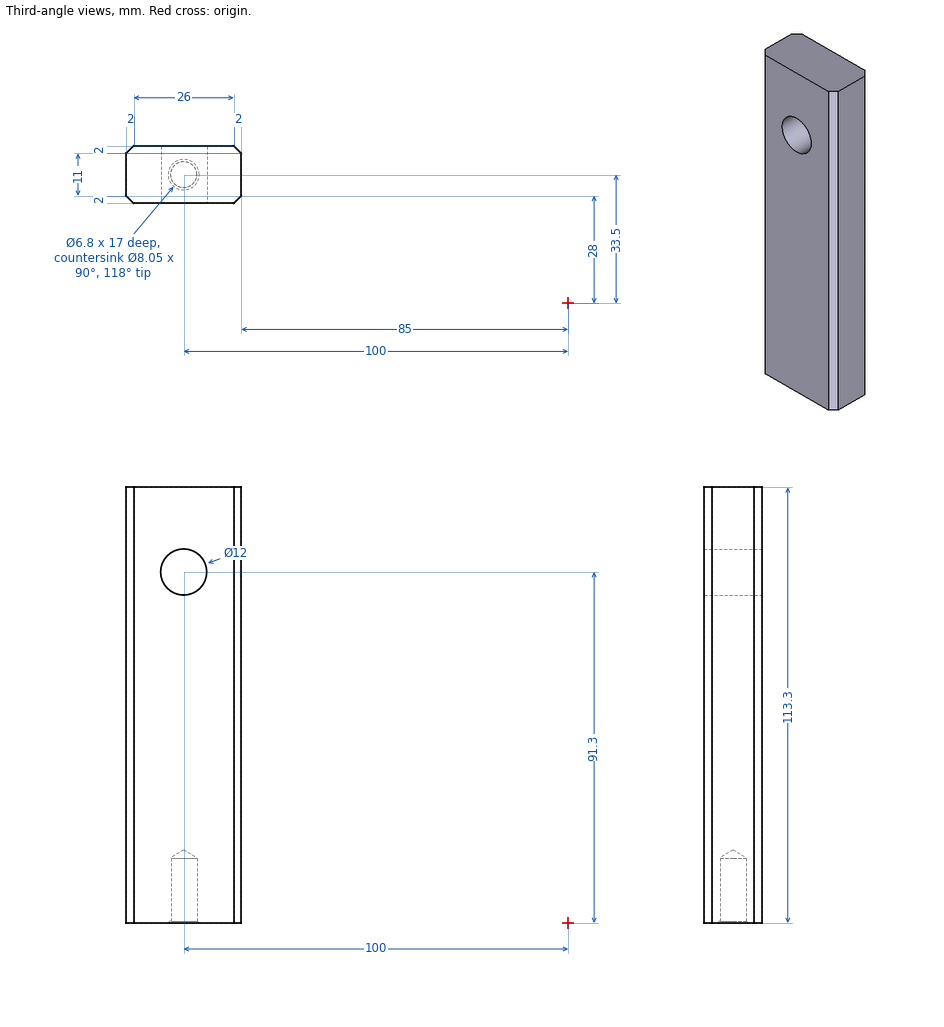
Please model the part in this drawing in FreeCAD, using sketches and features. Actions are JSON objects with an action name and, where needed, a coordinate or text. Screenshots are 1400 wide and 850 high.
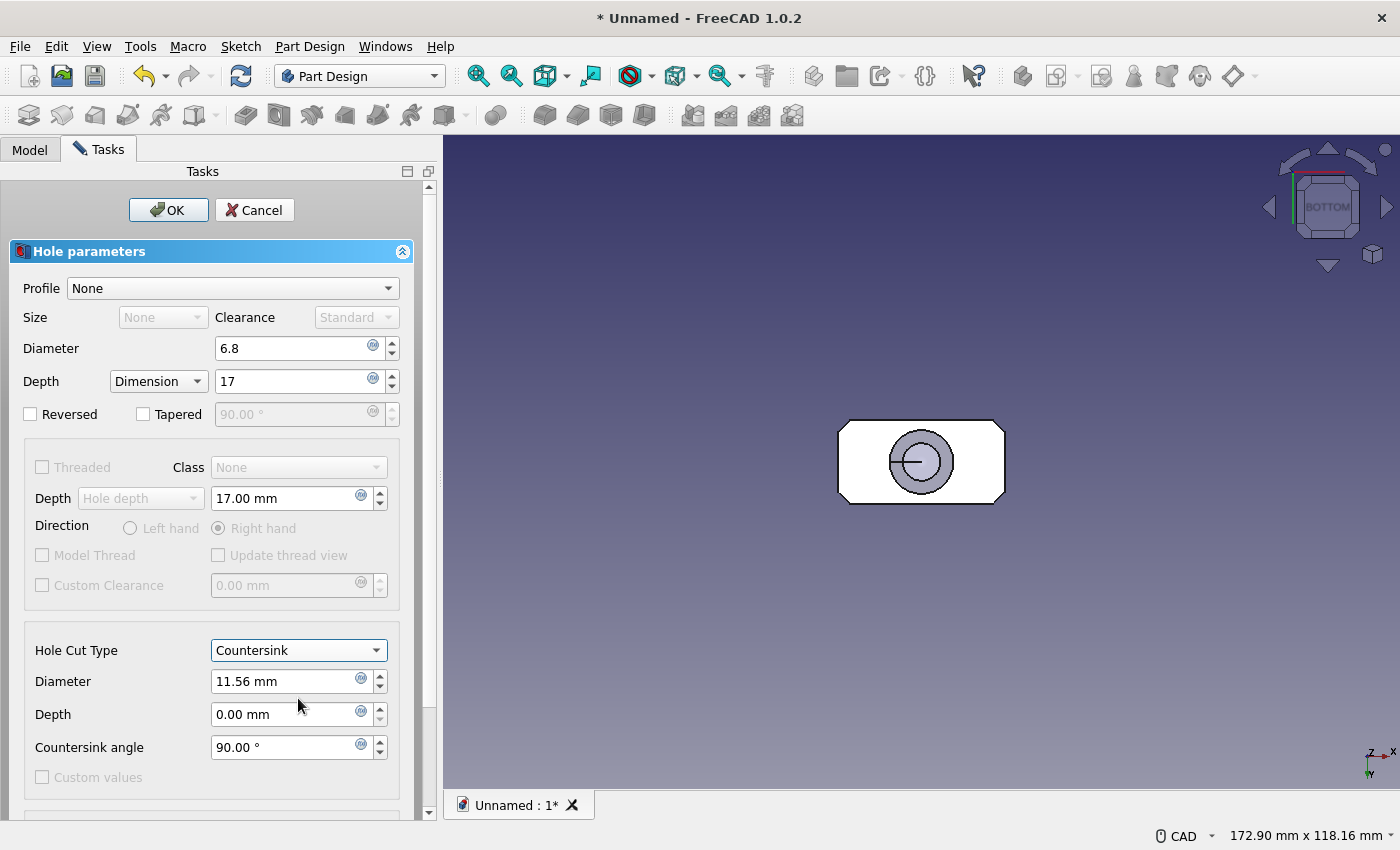
{"action": "triple_click", "coordinate": [292, 682]}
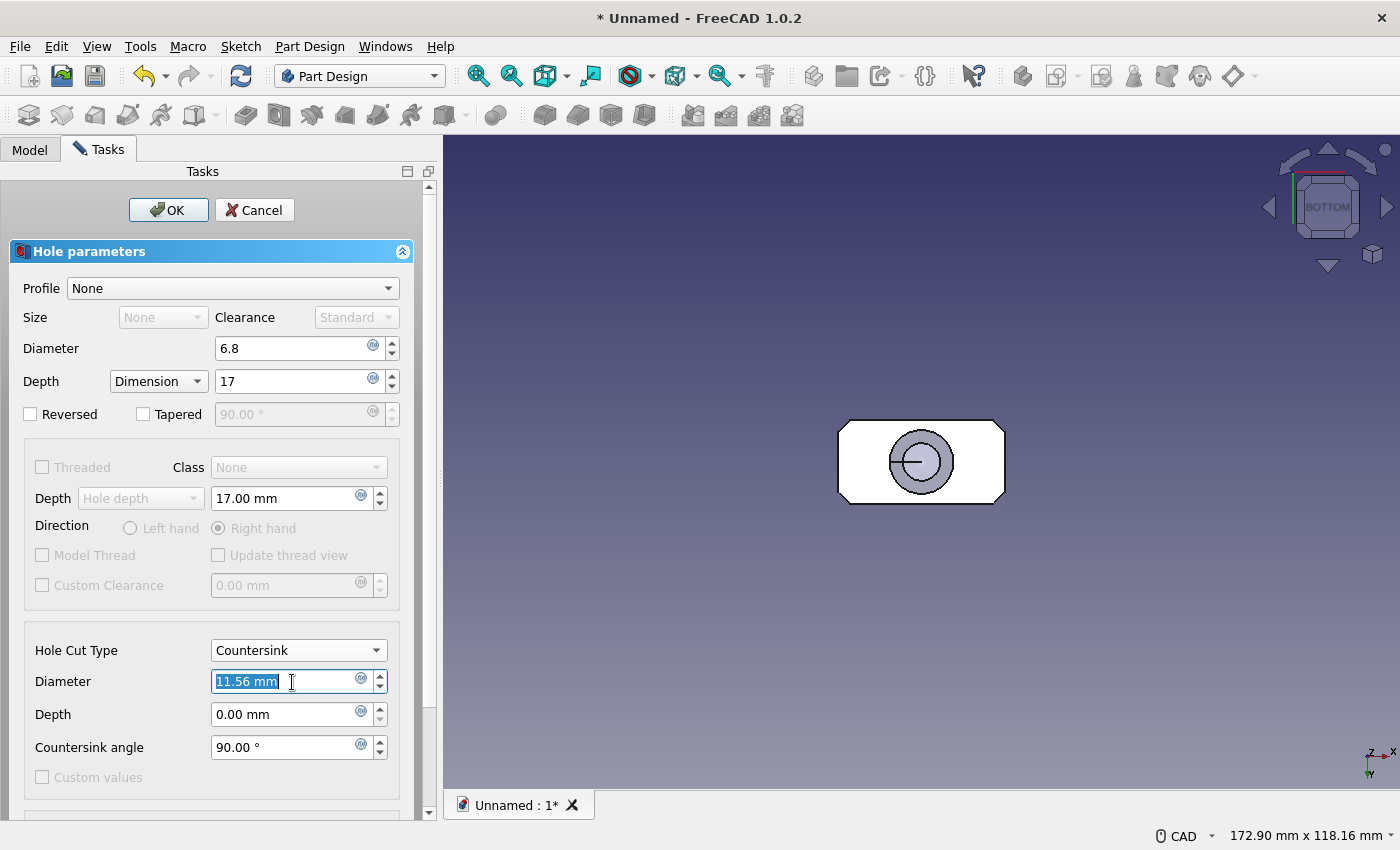
{"action": "type", "text": "8.05"}
{"action": "key", "text": "Tab"}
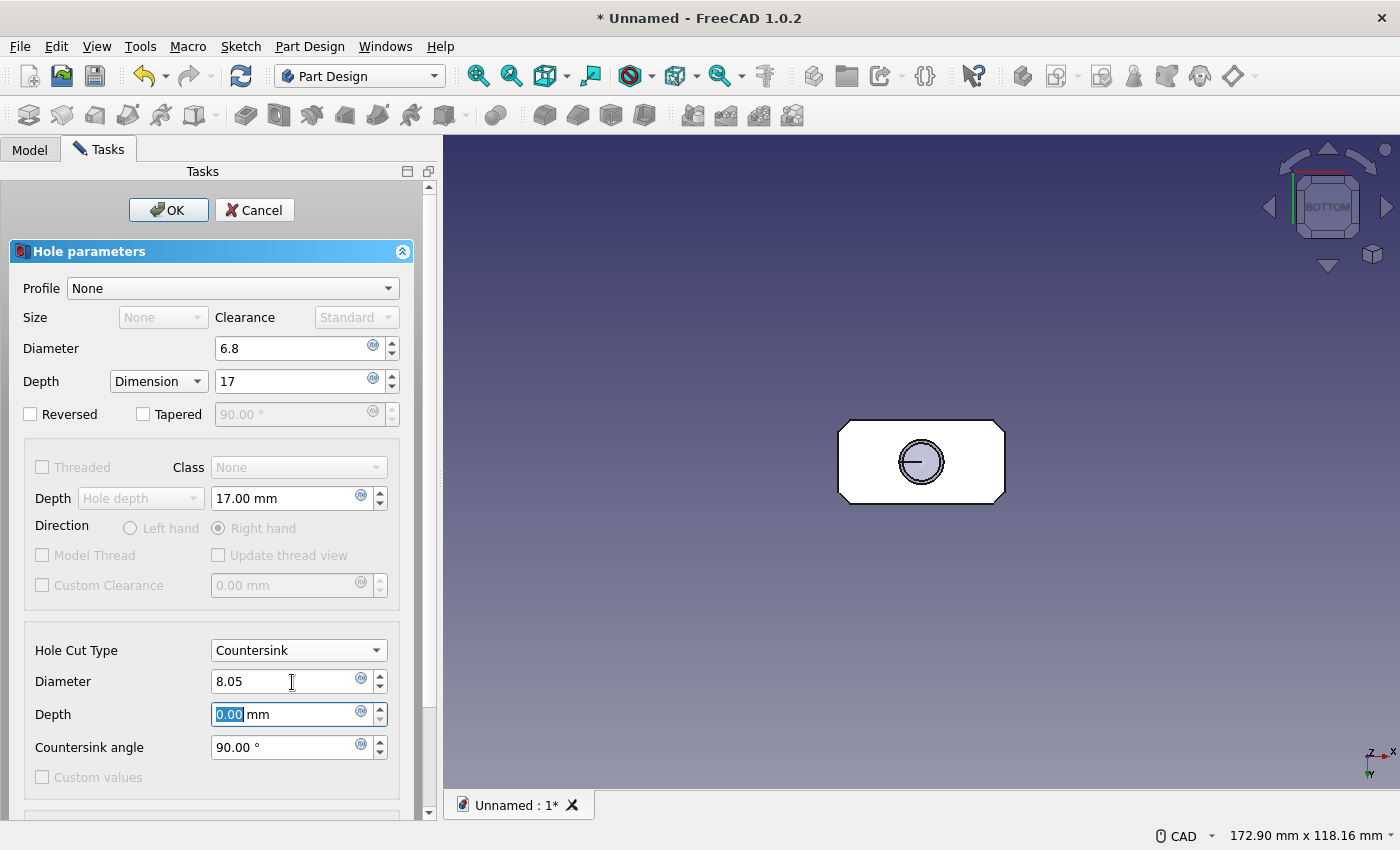
{"action": "left_click", "coordinate": [169, 210]}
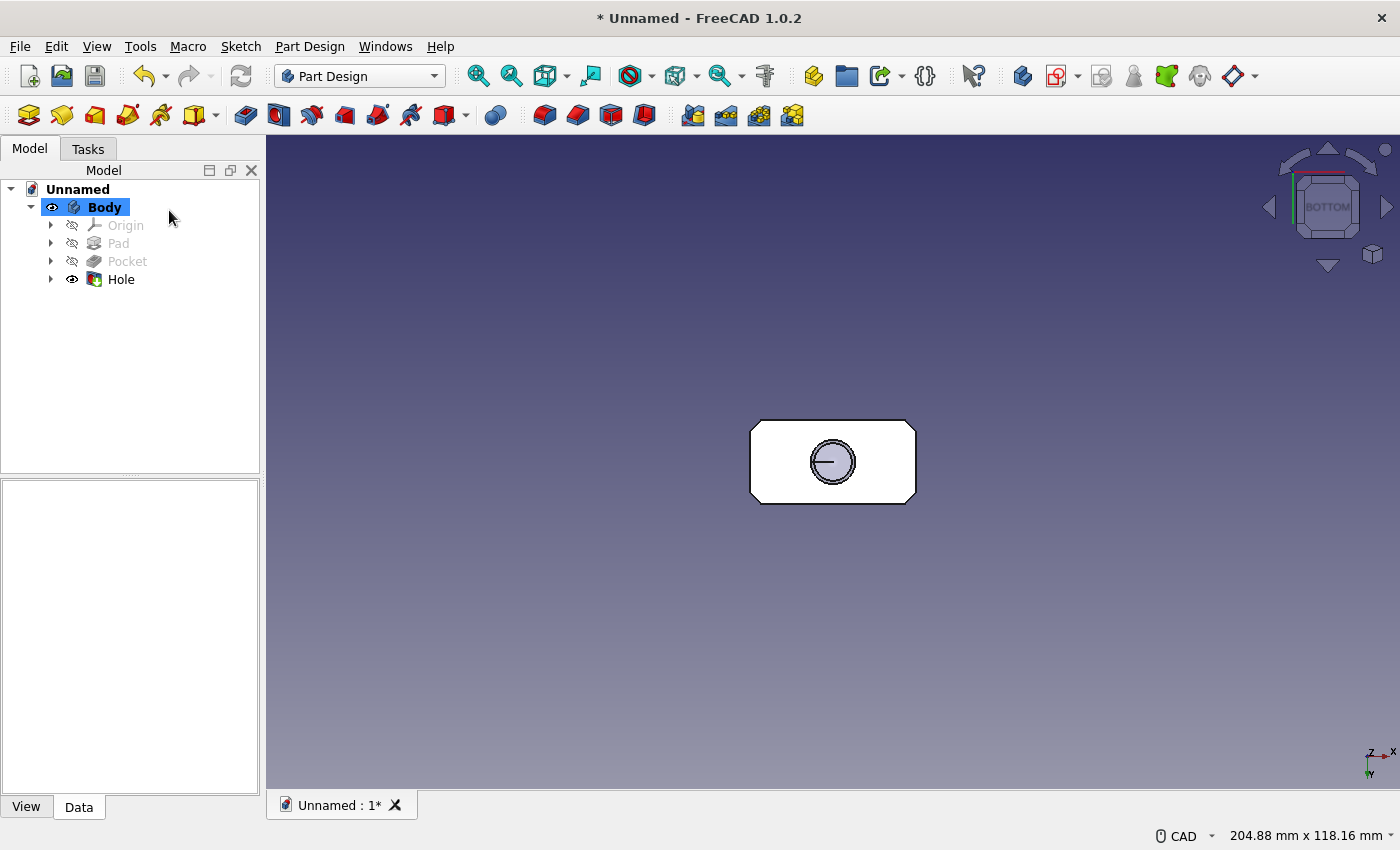
{"action": "key", "text": "0"}